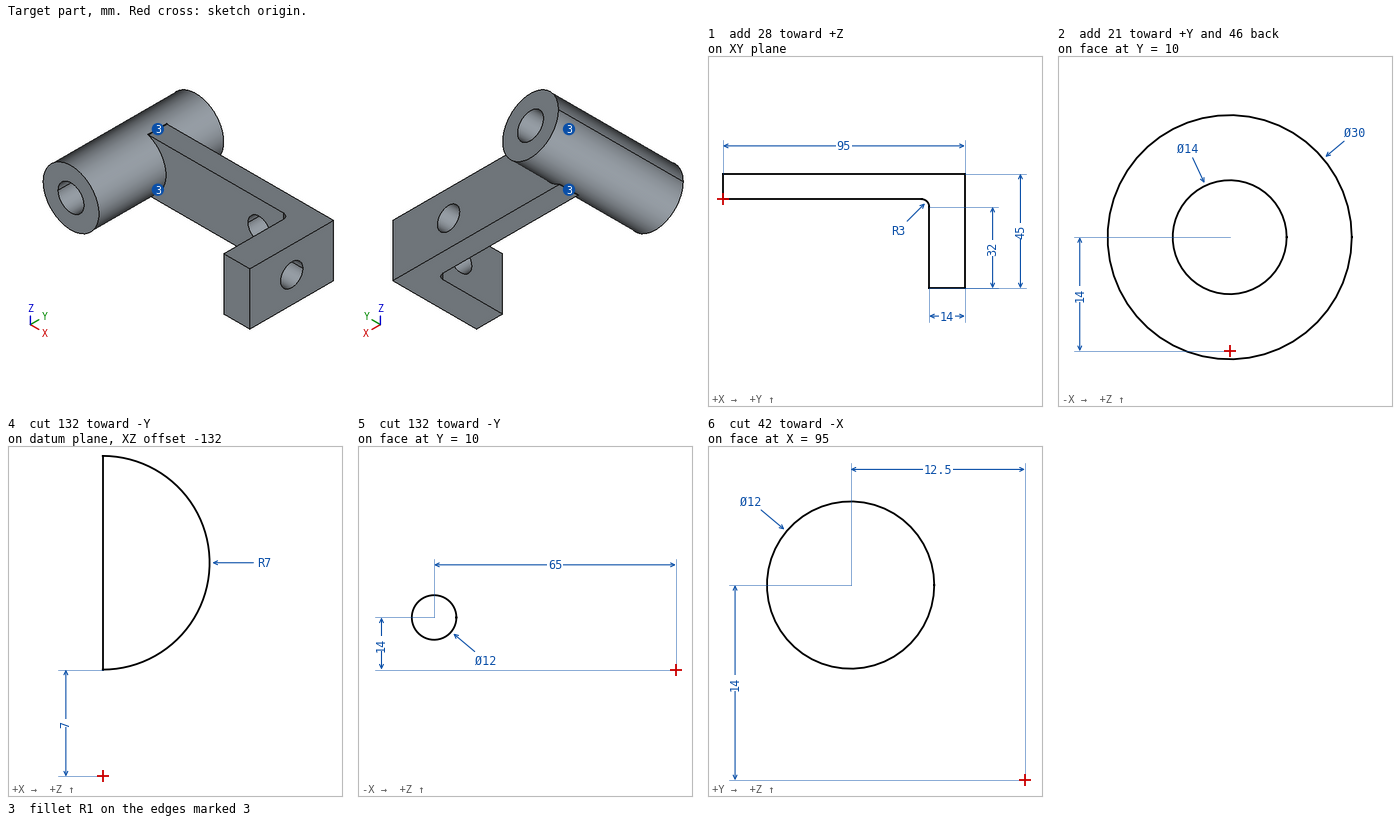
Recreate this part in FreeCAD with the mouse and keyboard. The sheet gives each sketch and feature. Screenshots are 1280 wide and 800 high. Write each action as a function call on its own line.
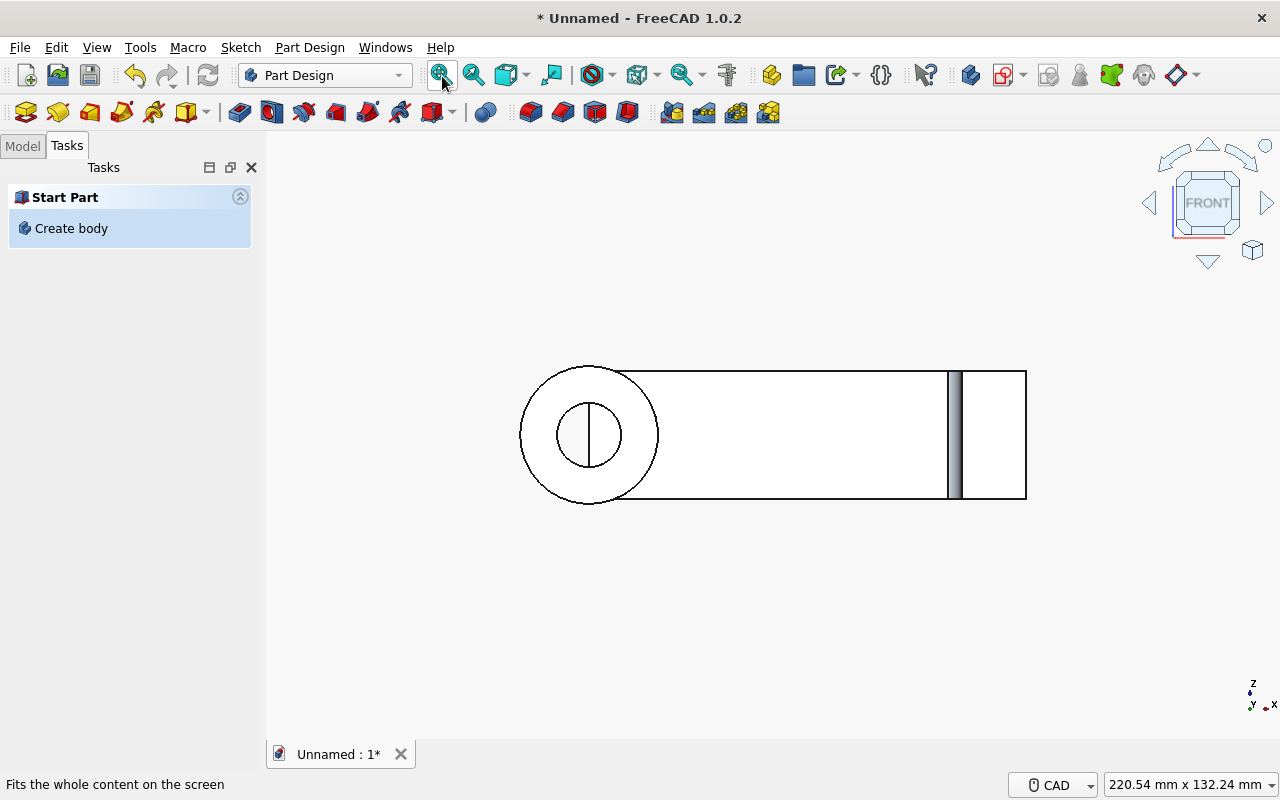
key(3)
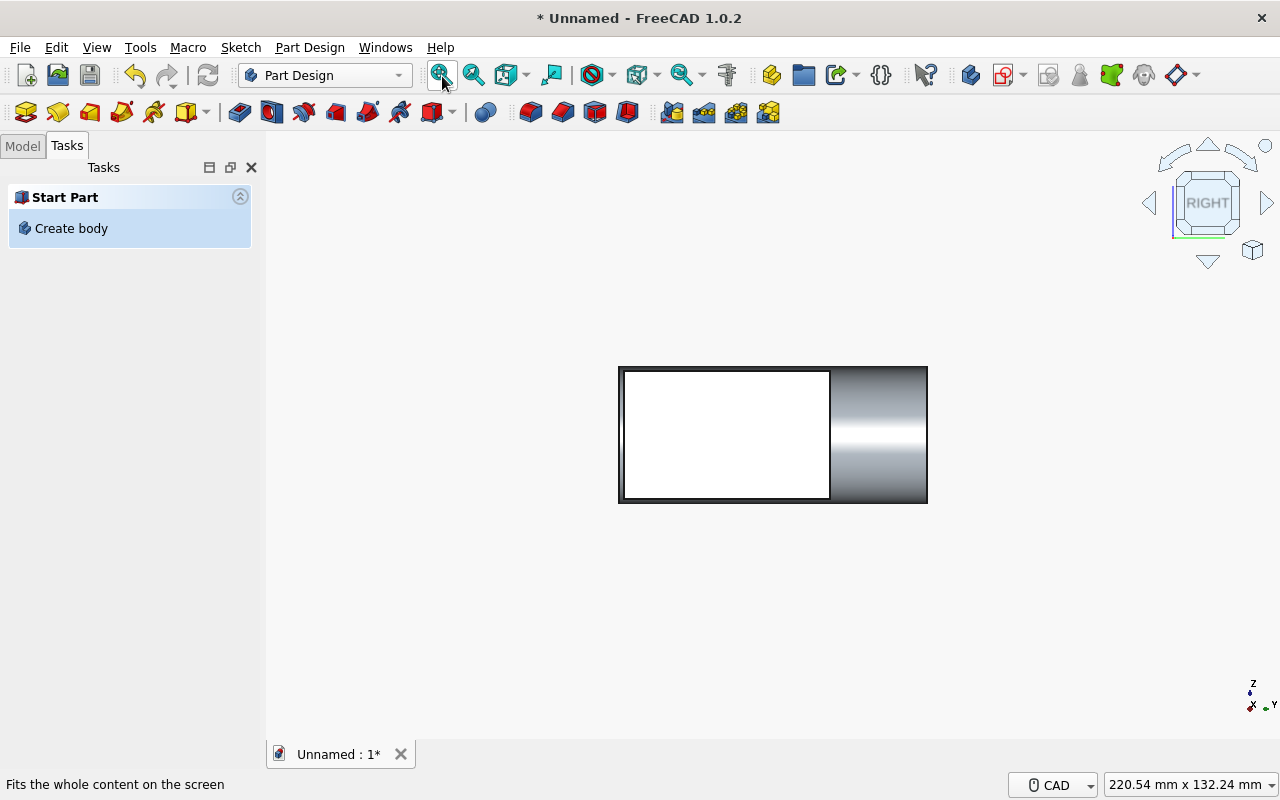
click(442, 76)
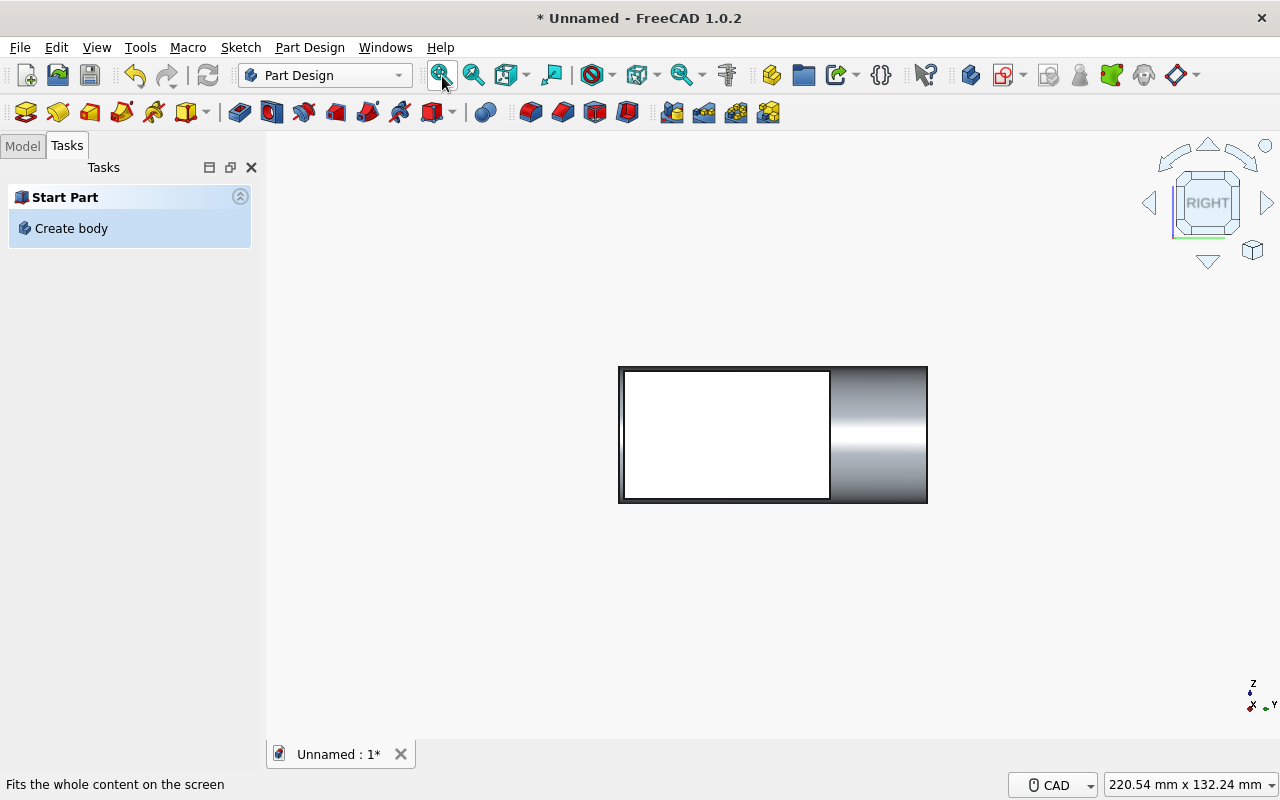
key(5)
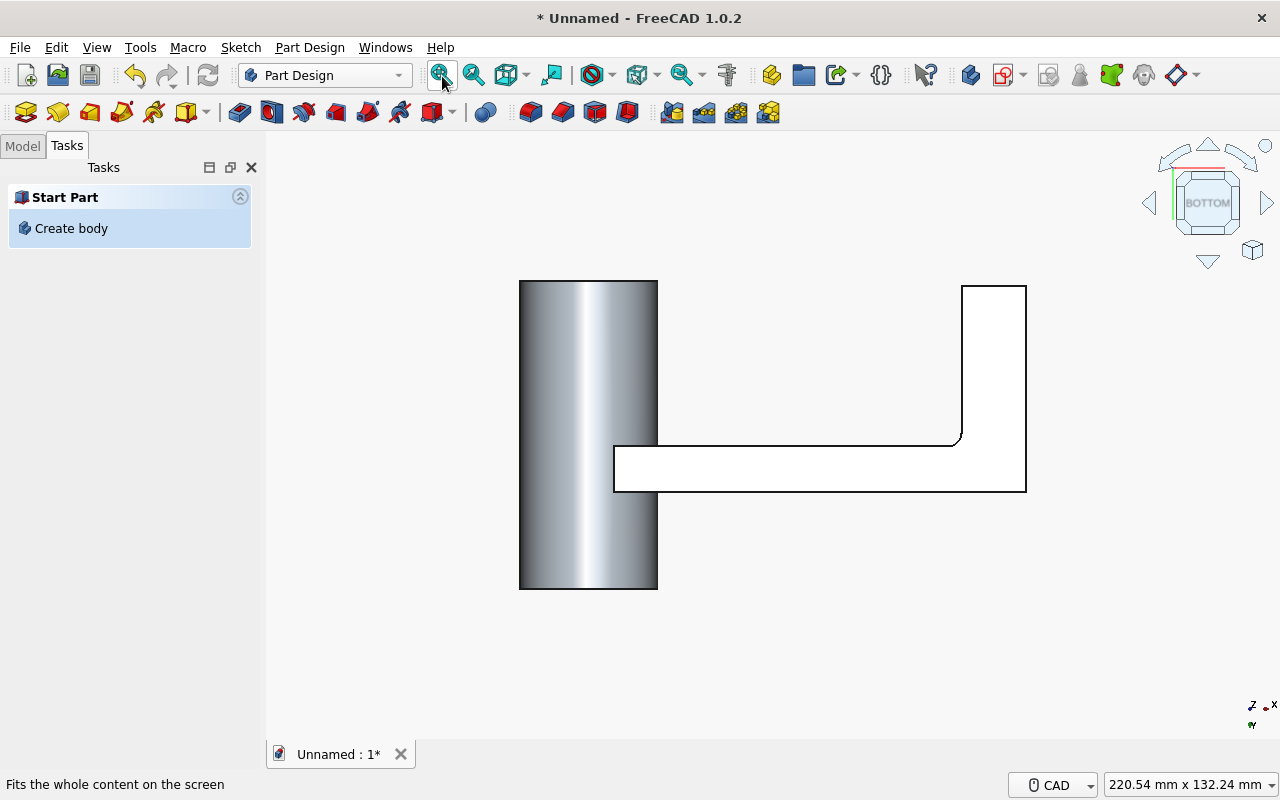
key(4)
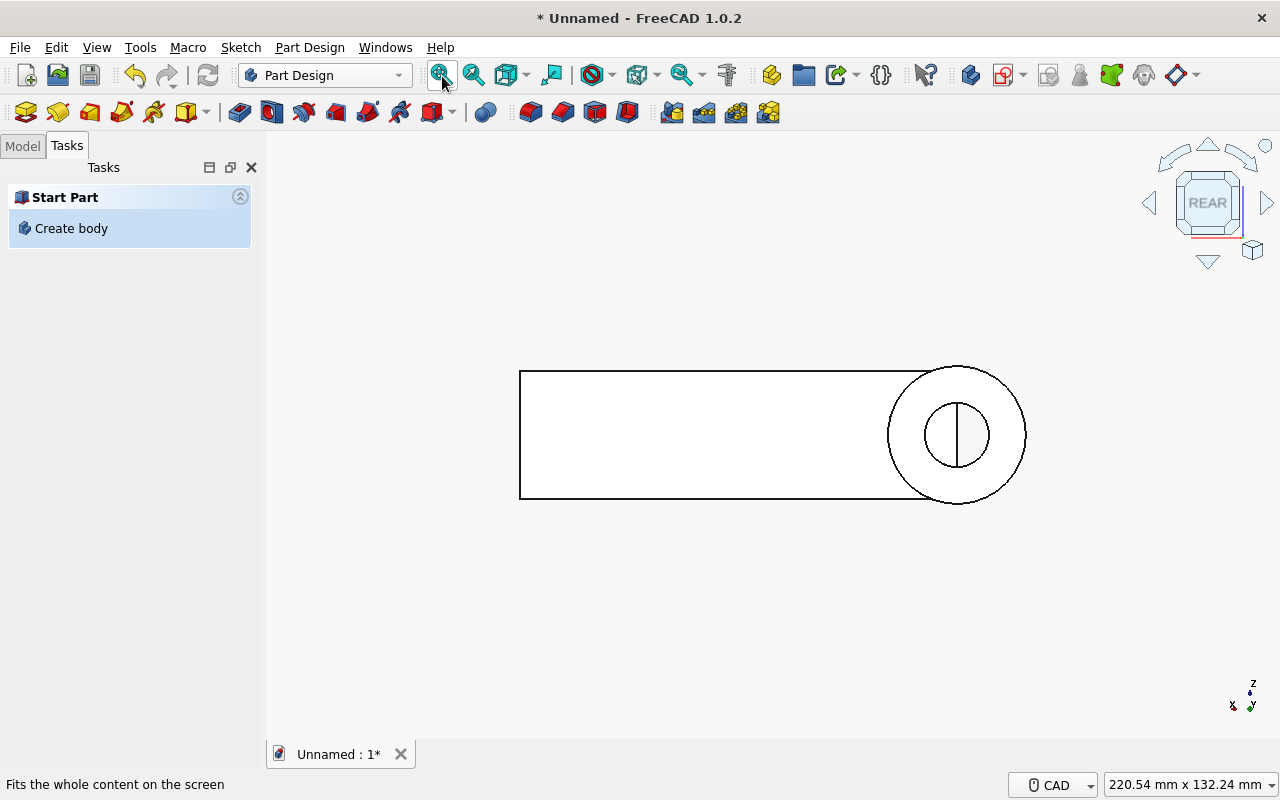
key(6)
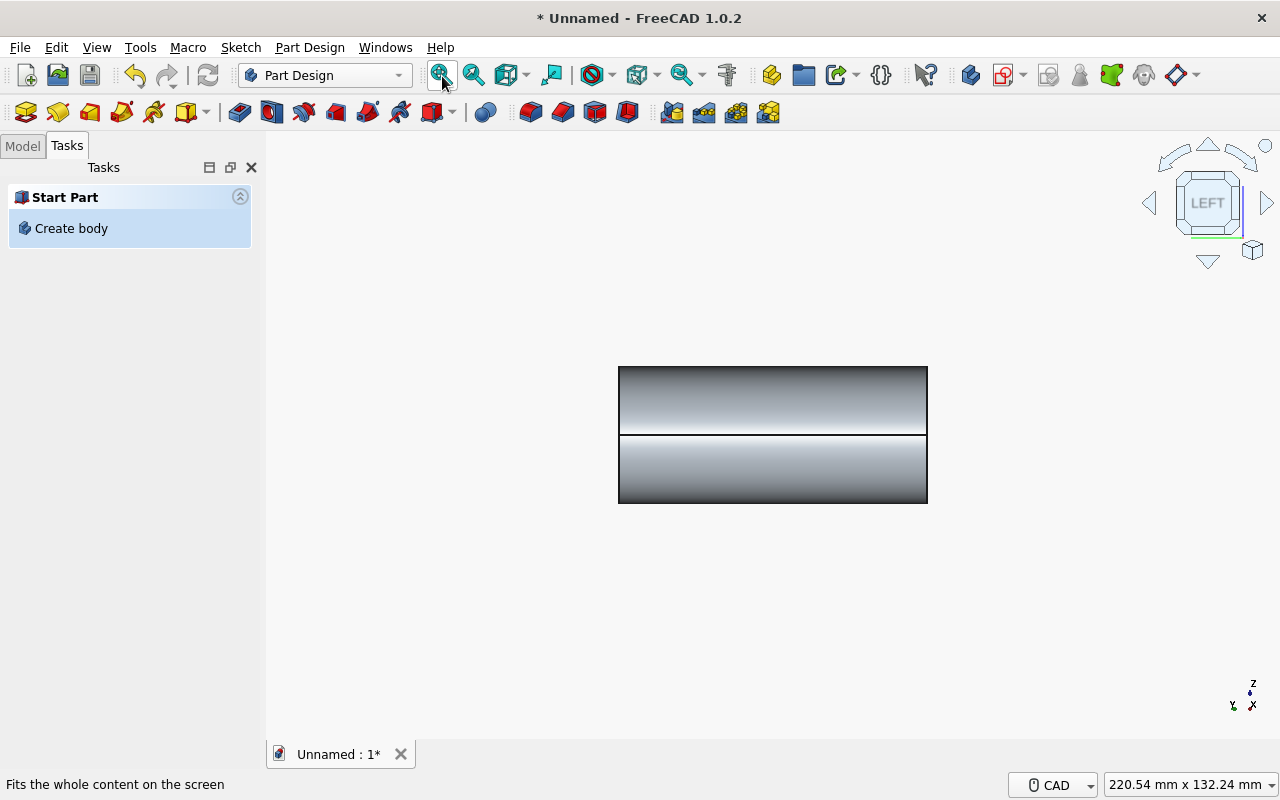
click(442, 76)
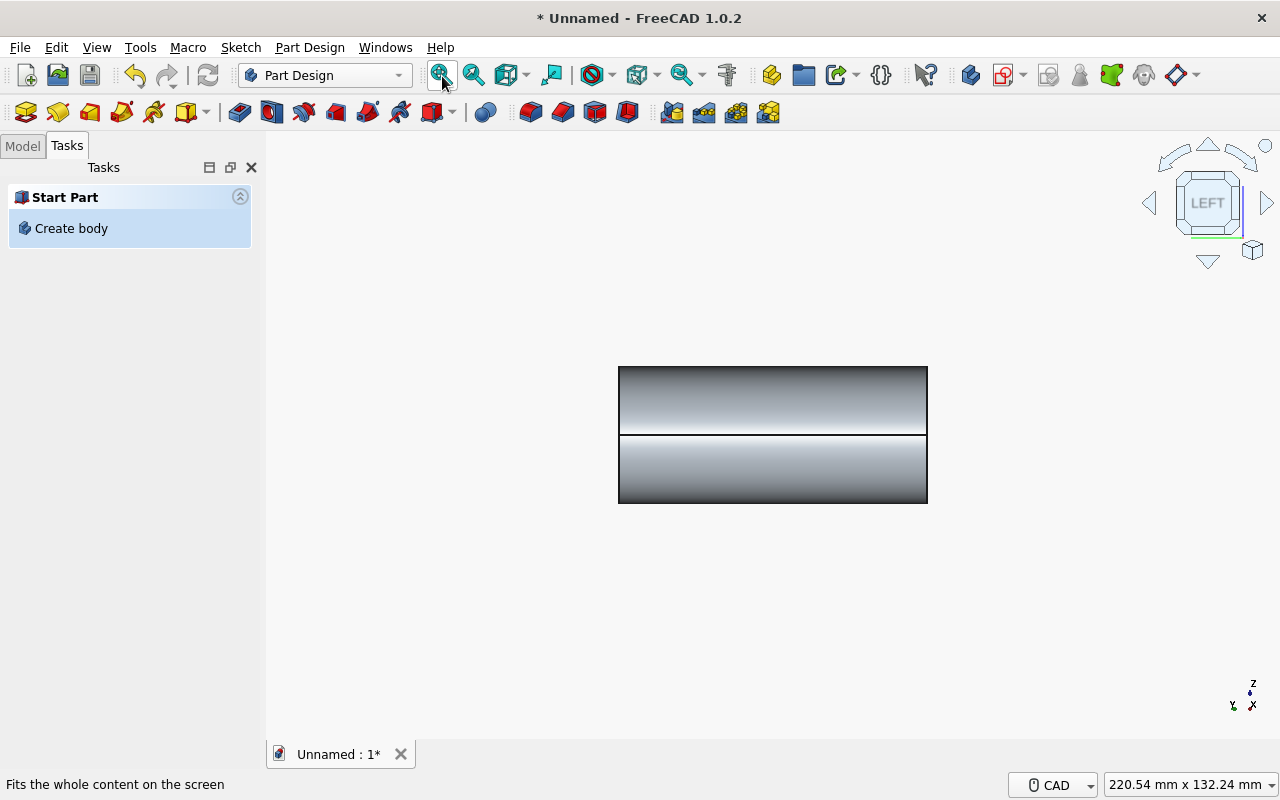
key(v)
key(3)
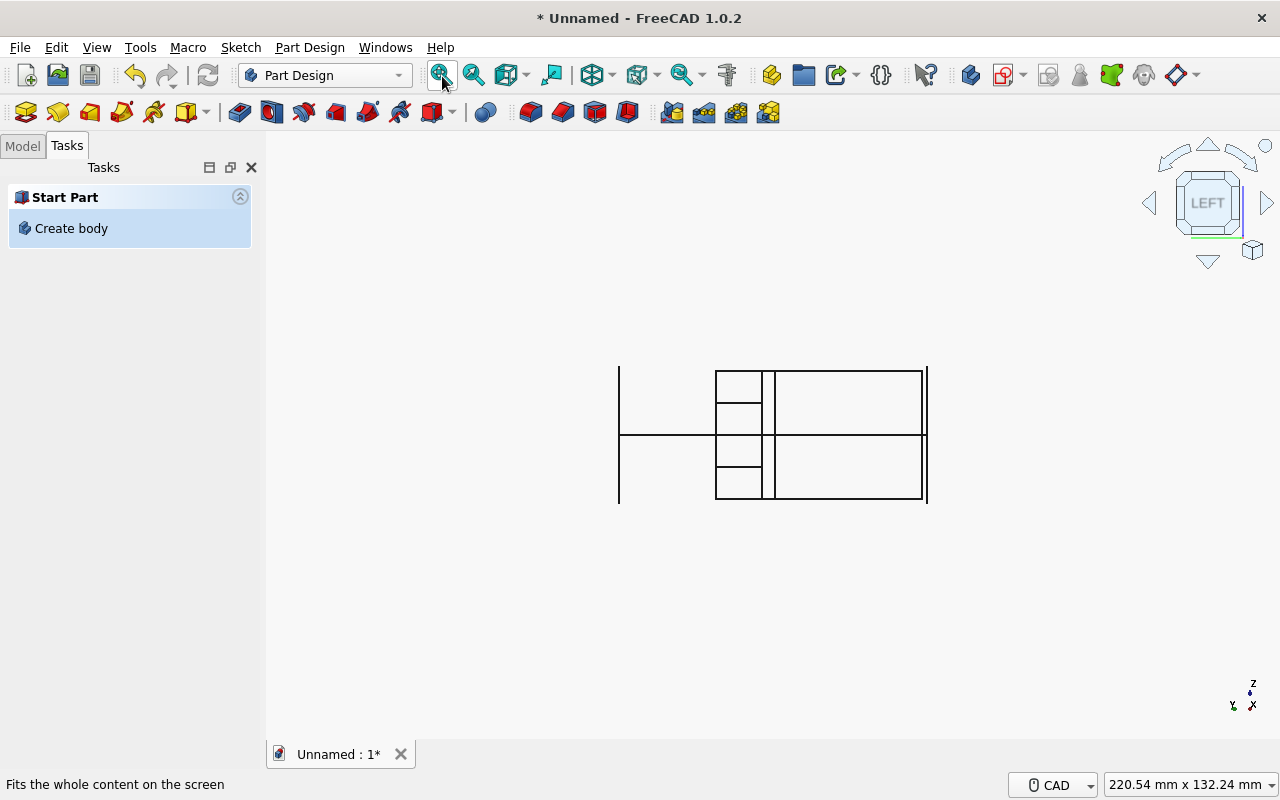
key(0)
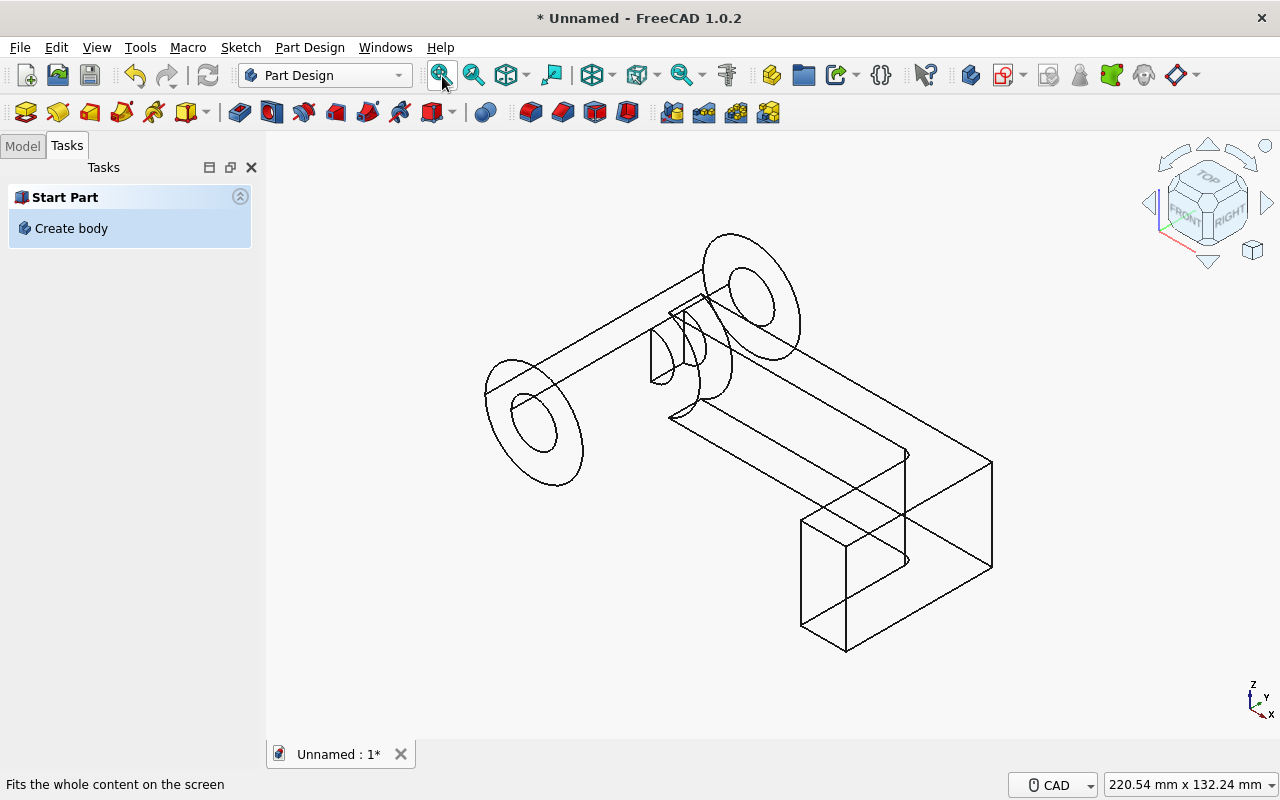
click(685, 302)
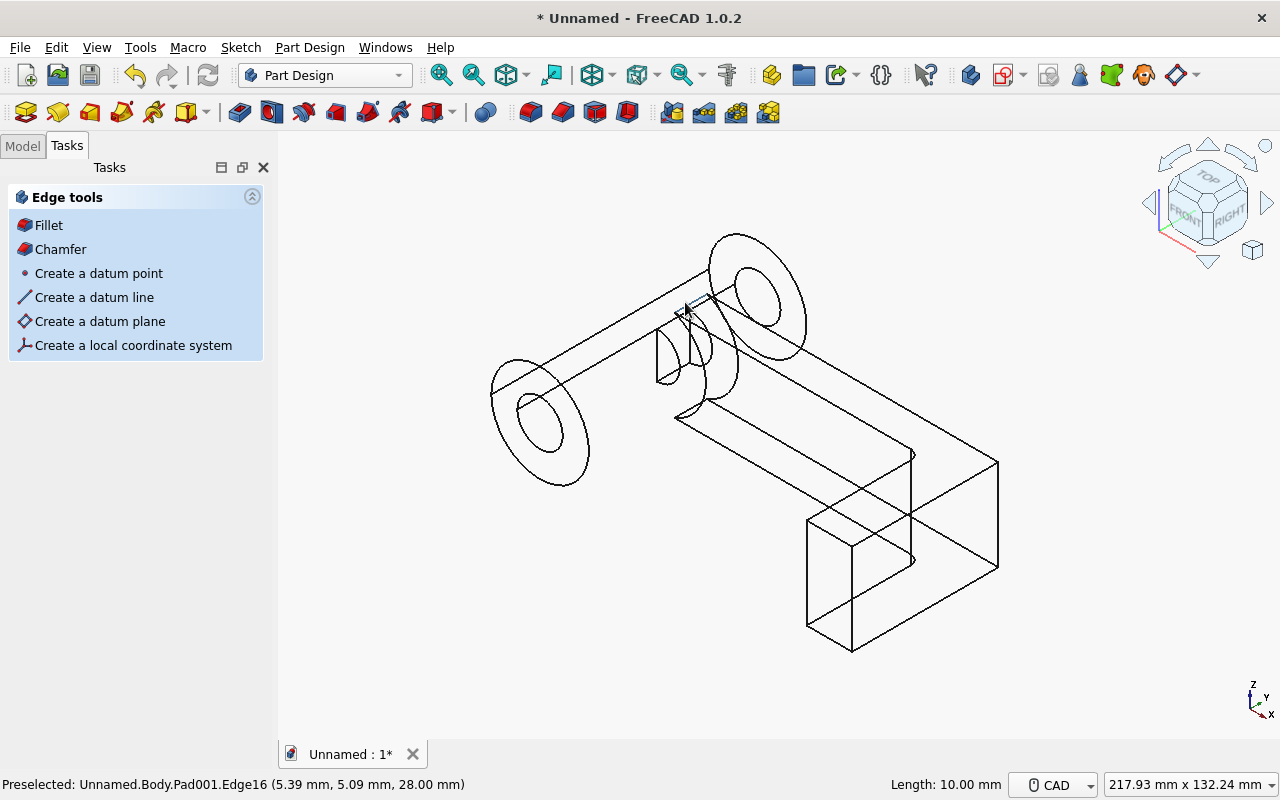
scroll(691, 408, up, 6)